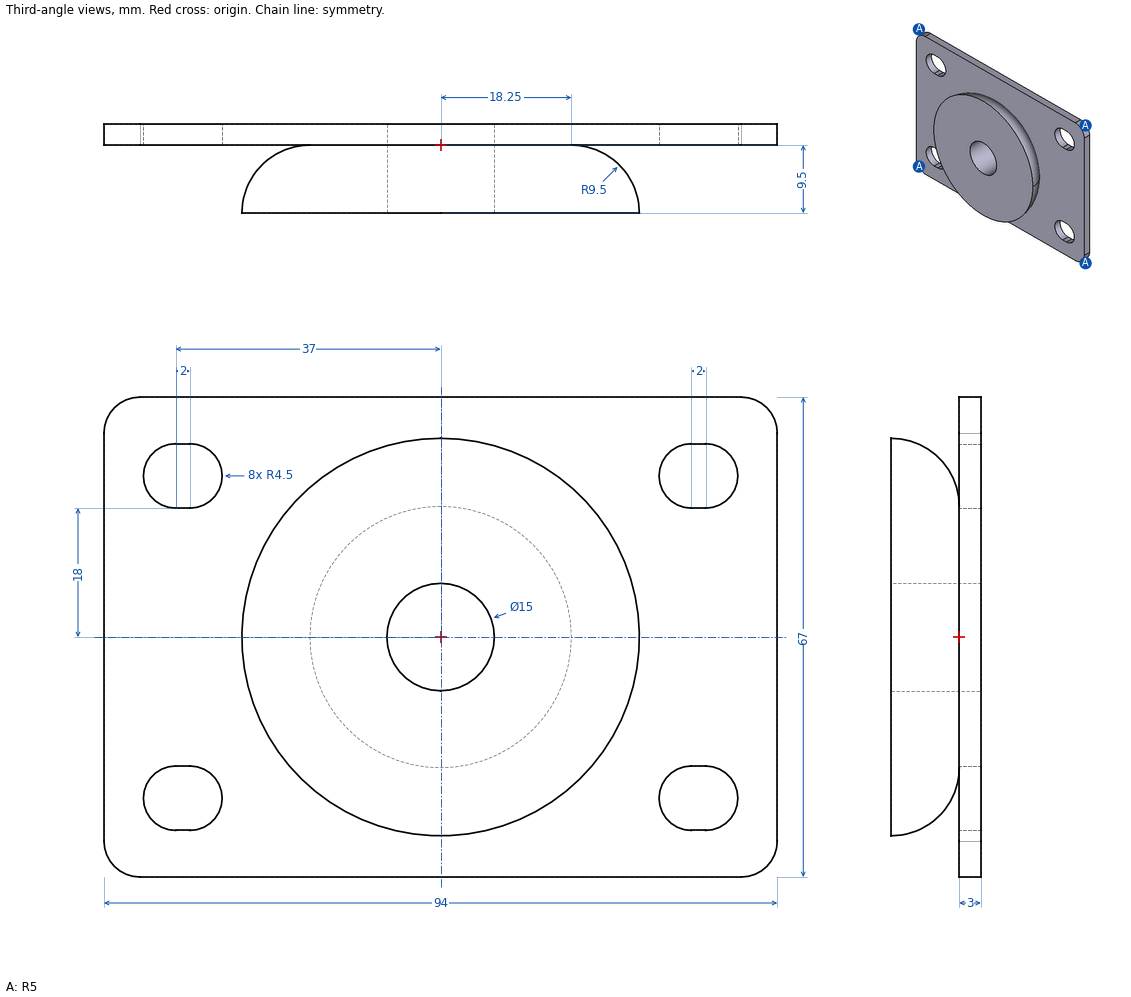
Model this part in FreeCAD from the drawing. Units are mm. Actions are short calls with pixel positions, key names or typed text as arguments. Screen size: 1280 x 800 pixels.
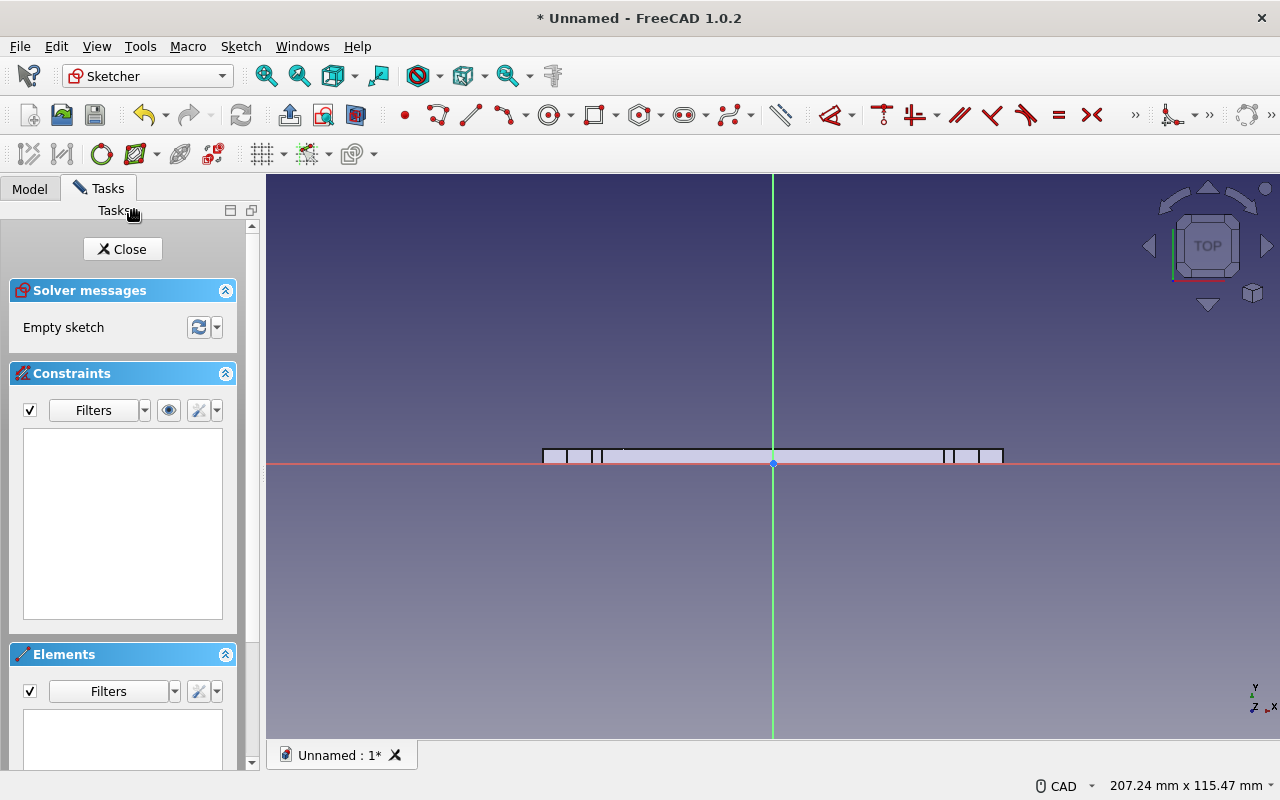
scroll(886, 497, up, 7)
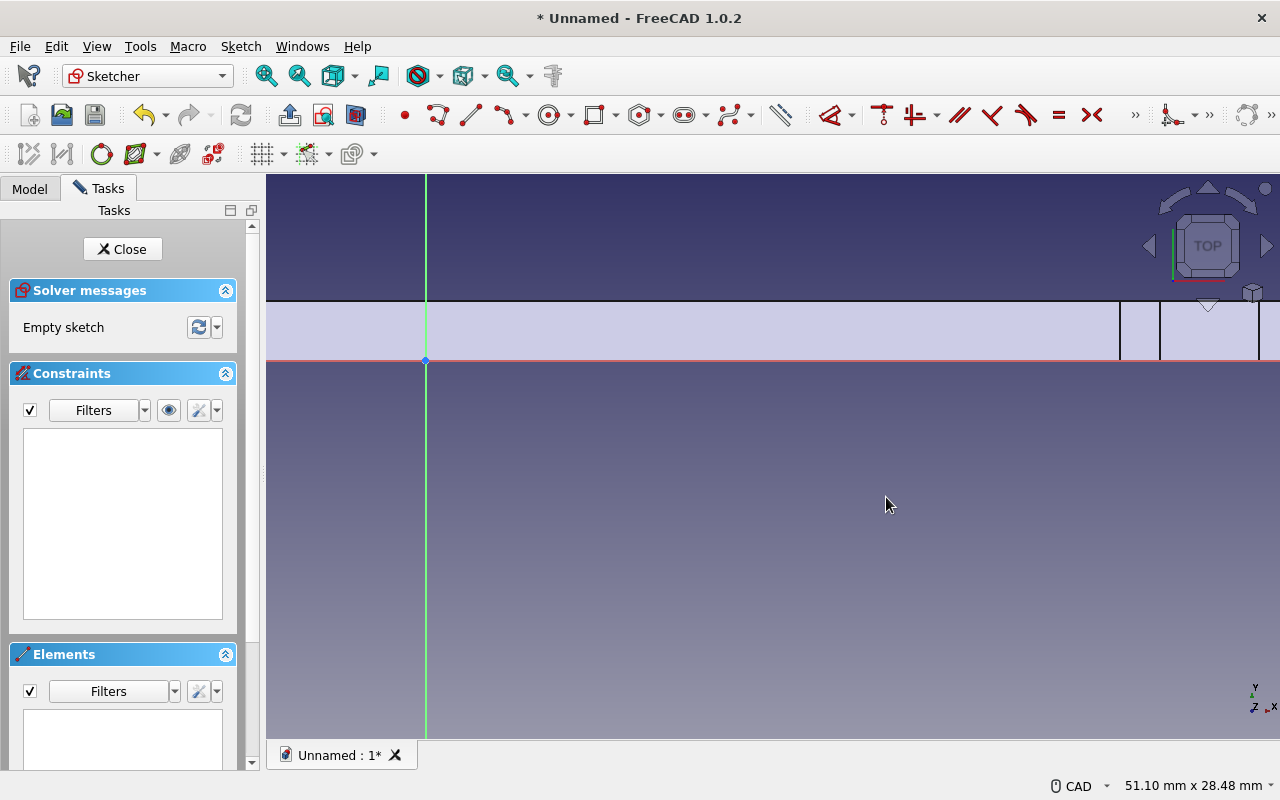
key(g)
key(m)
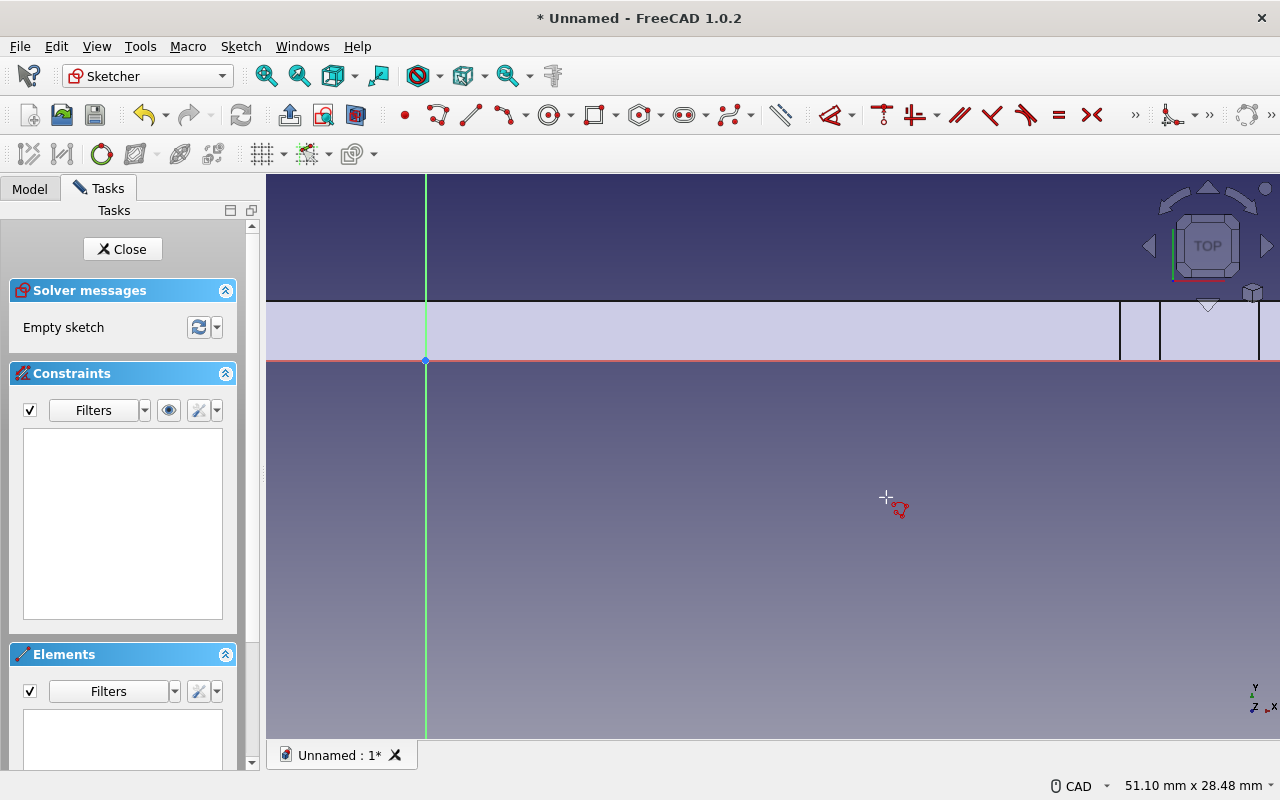
click(788, 361)
click(426, 361)
click(435, 549)
click(977, 549)
right_click(977, 549)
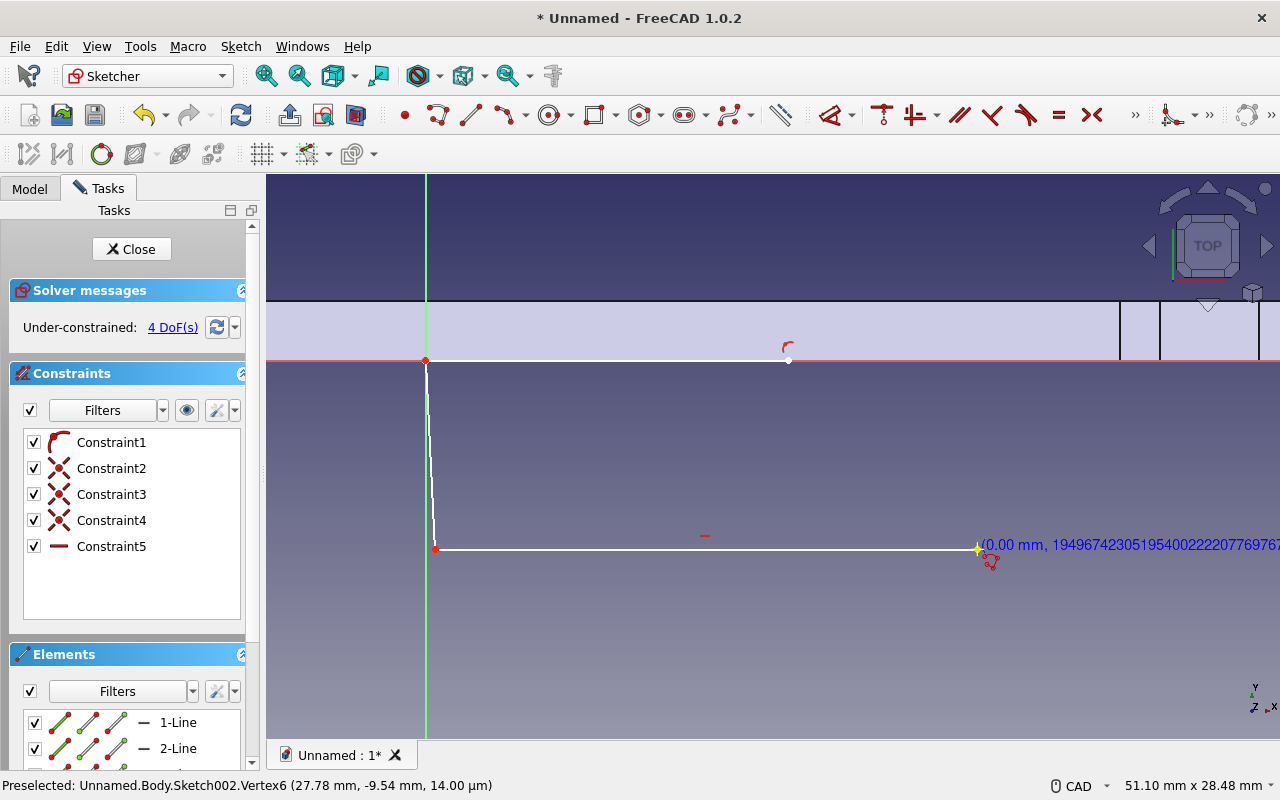
click(504, 116)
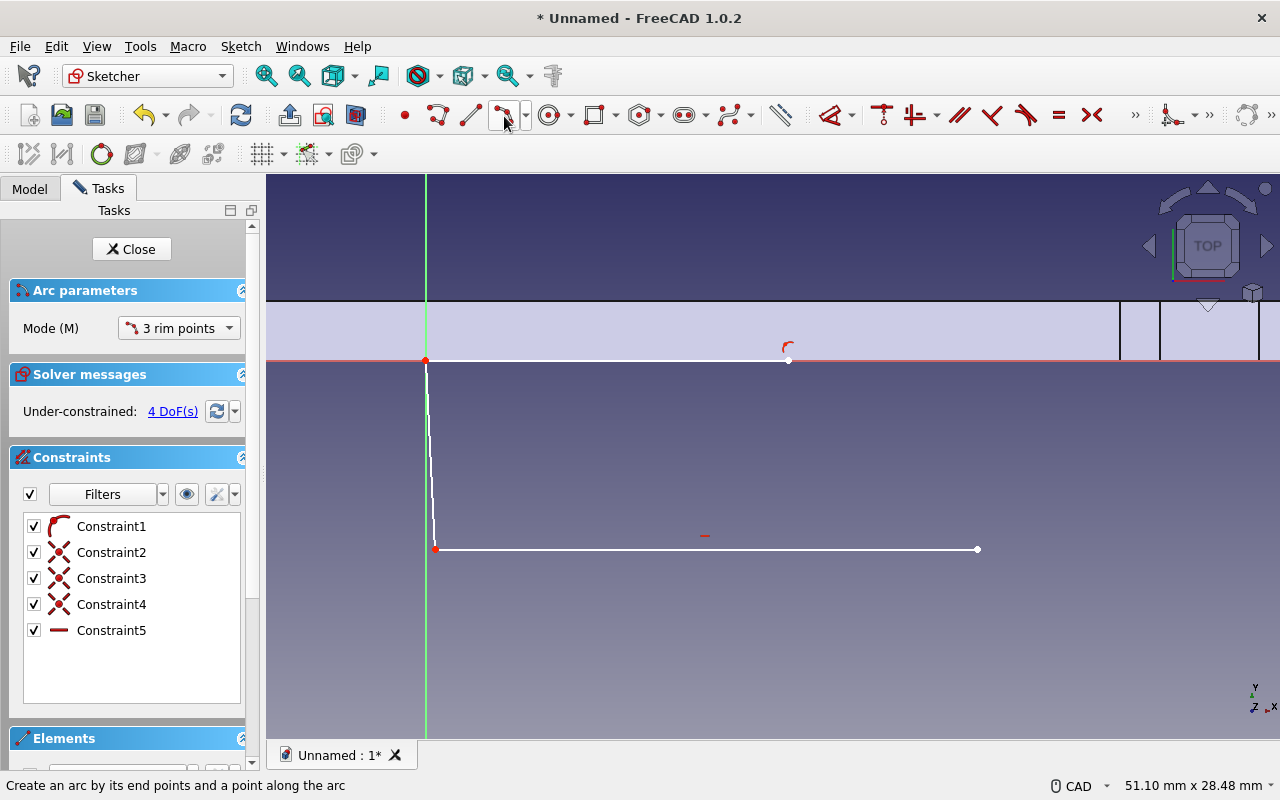
click(977, 550)
click(788, 361)
click(921, 416)
key(Escape)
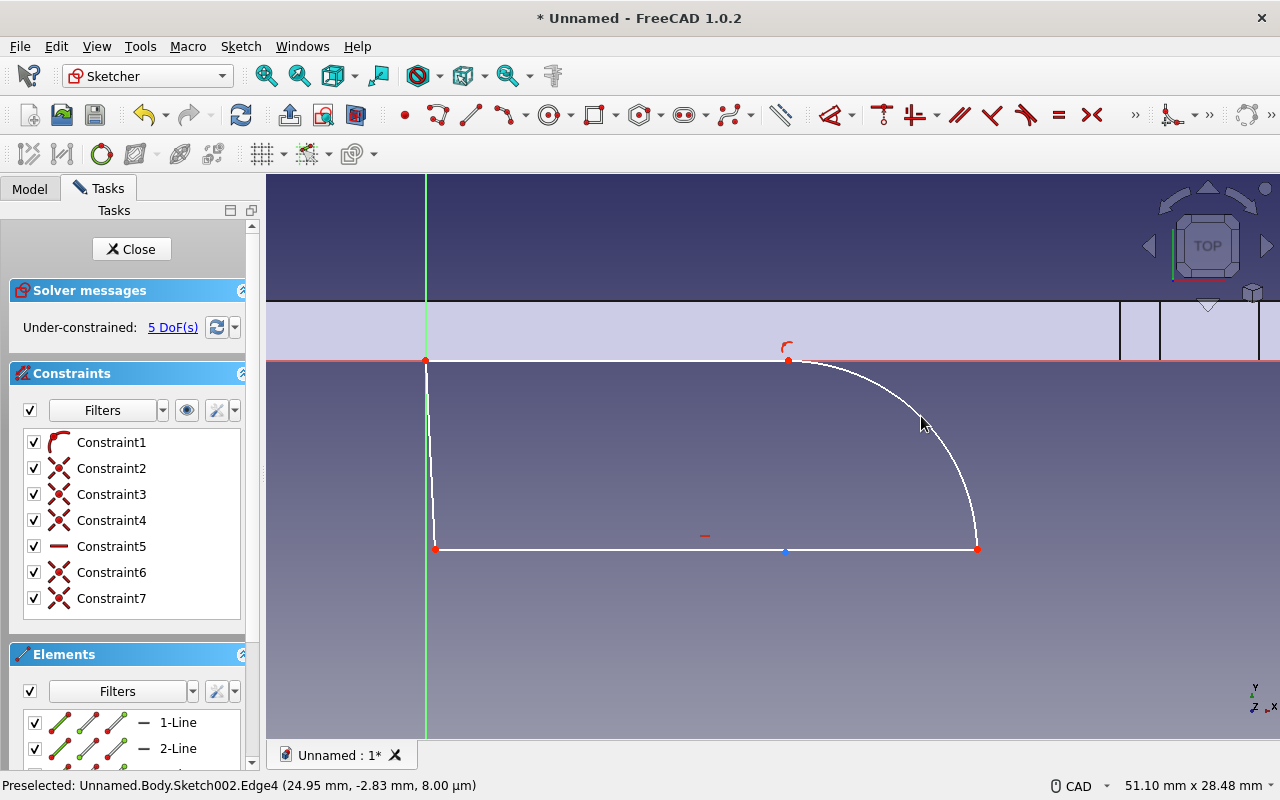
click(679, 361)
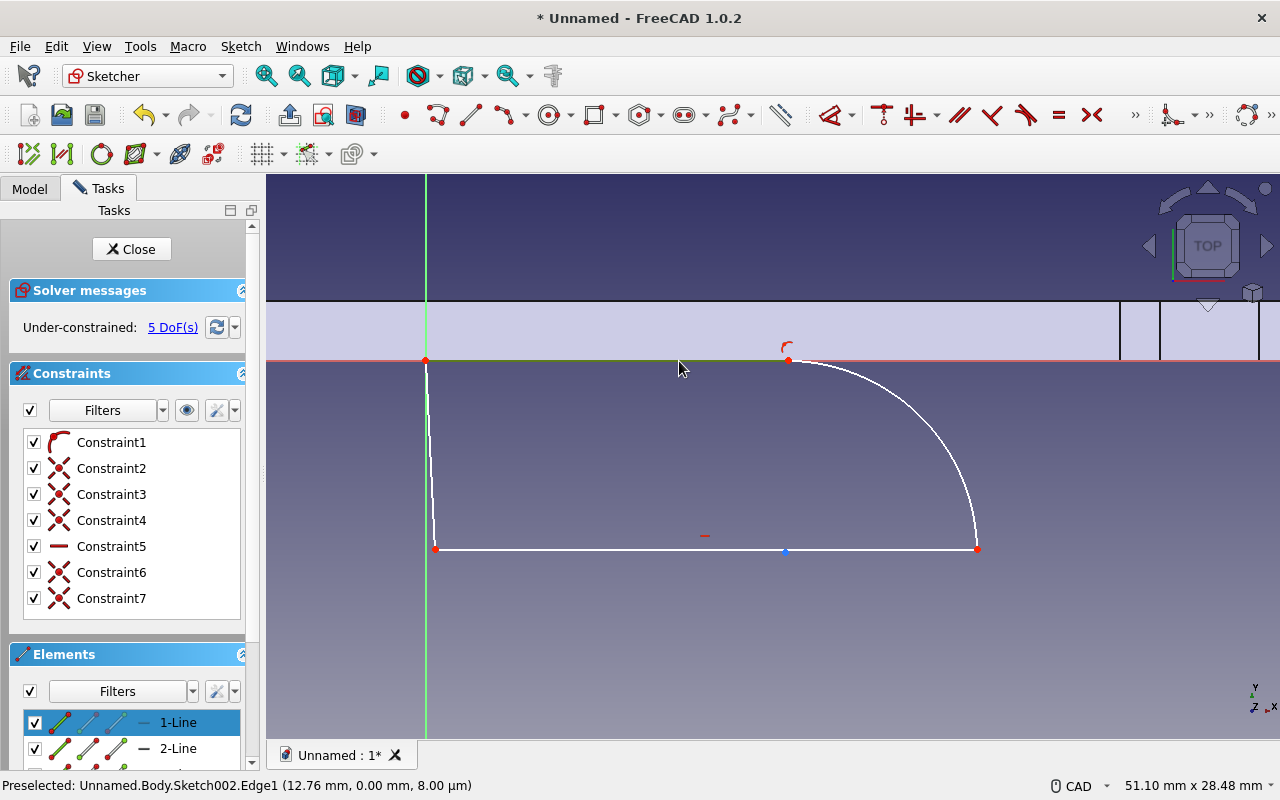
click(956, 465)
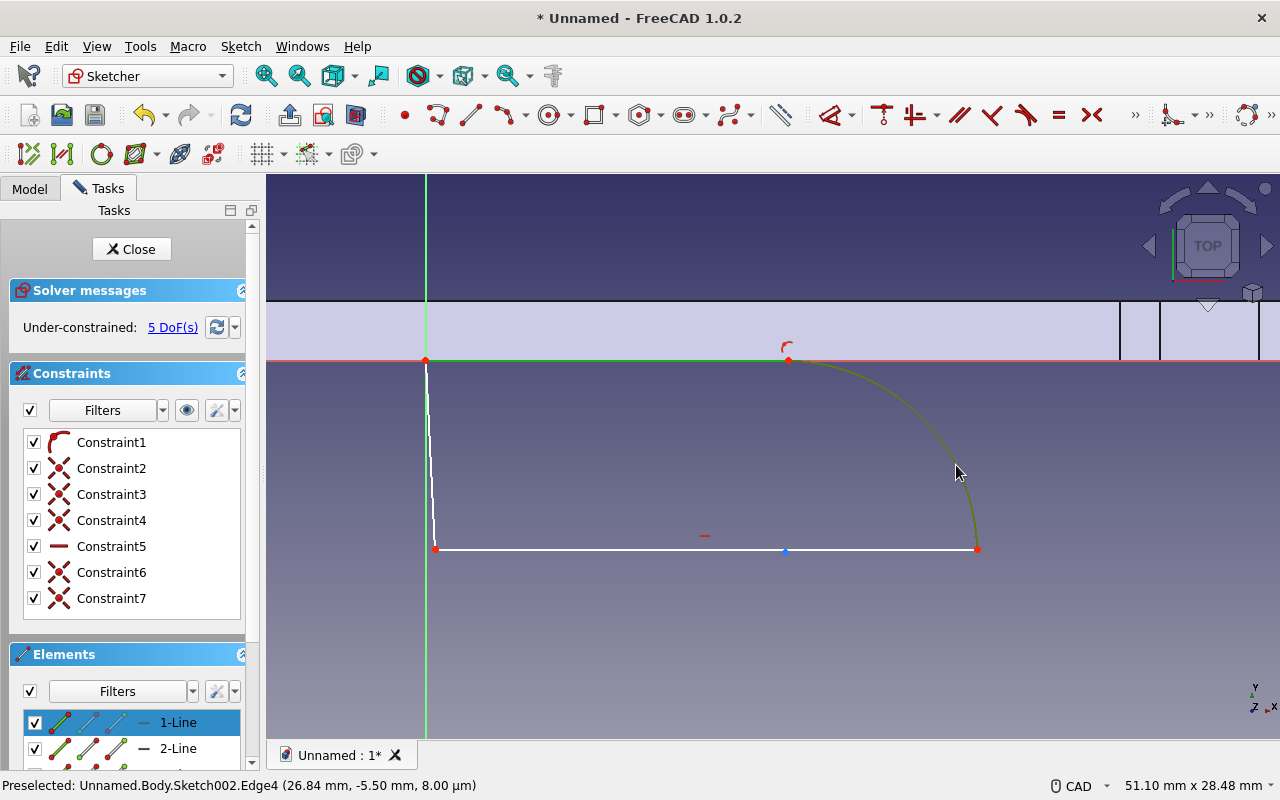
key(t)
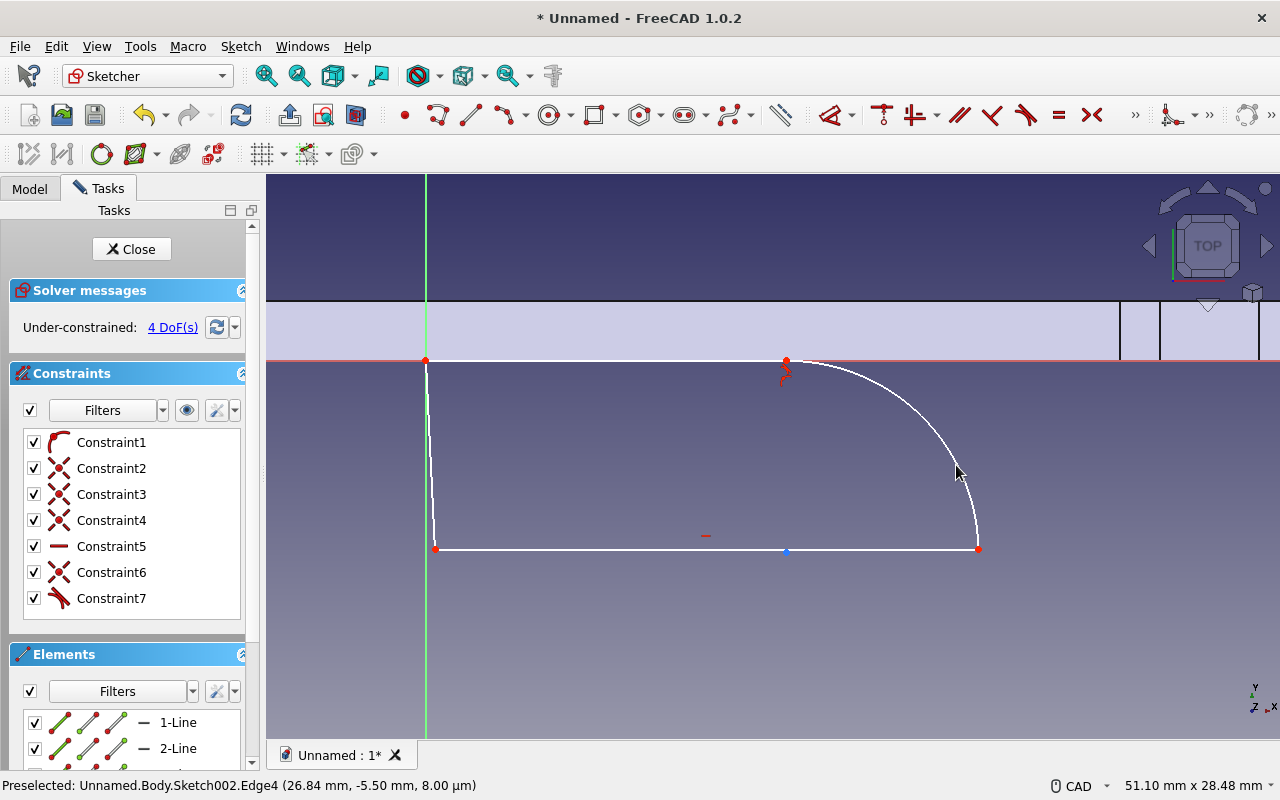
click(429, 418)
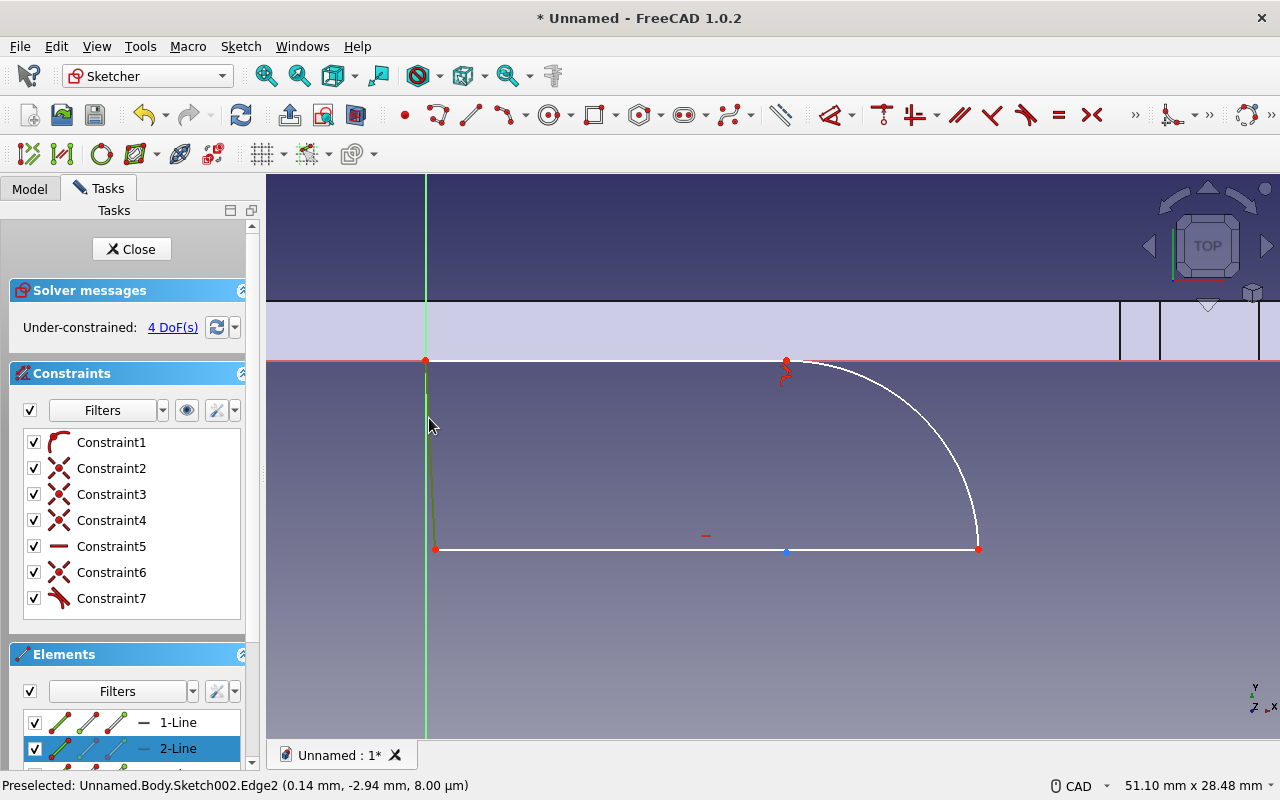
click(936, 116)